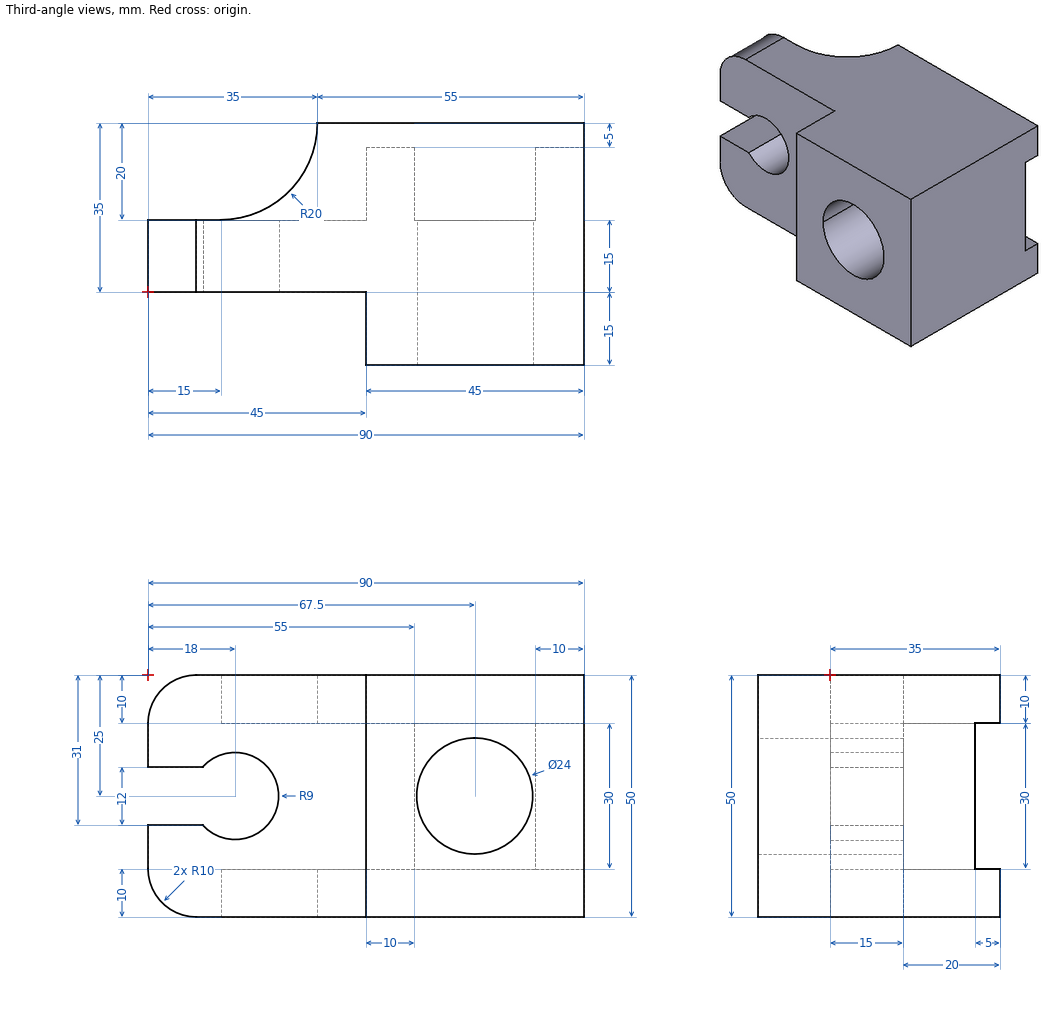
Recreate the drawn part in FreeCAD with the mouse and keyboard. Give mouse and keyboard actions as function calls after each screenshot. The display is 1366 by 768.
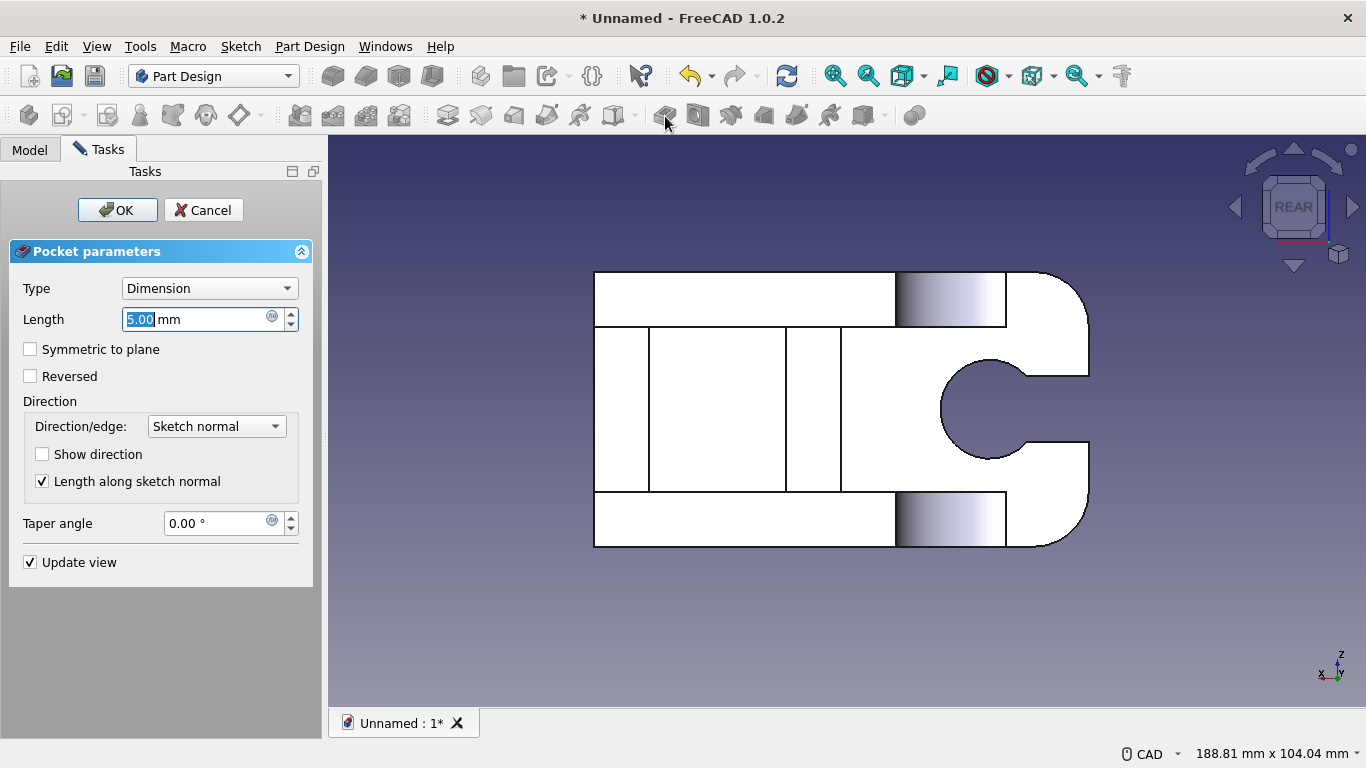
text(5)
key(Tab)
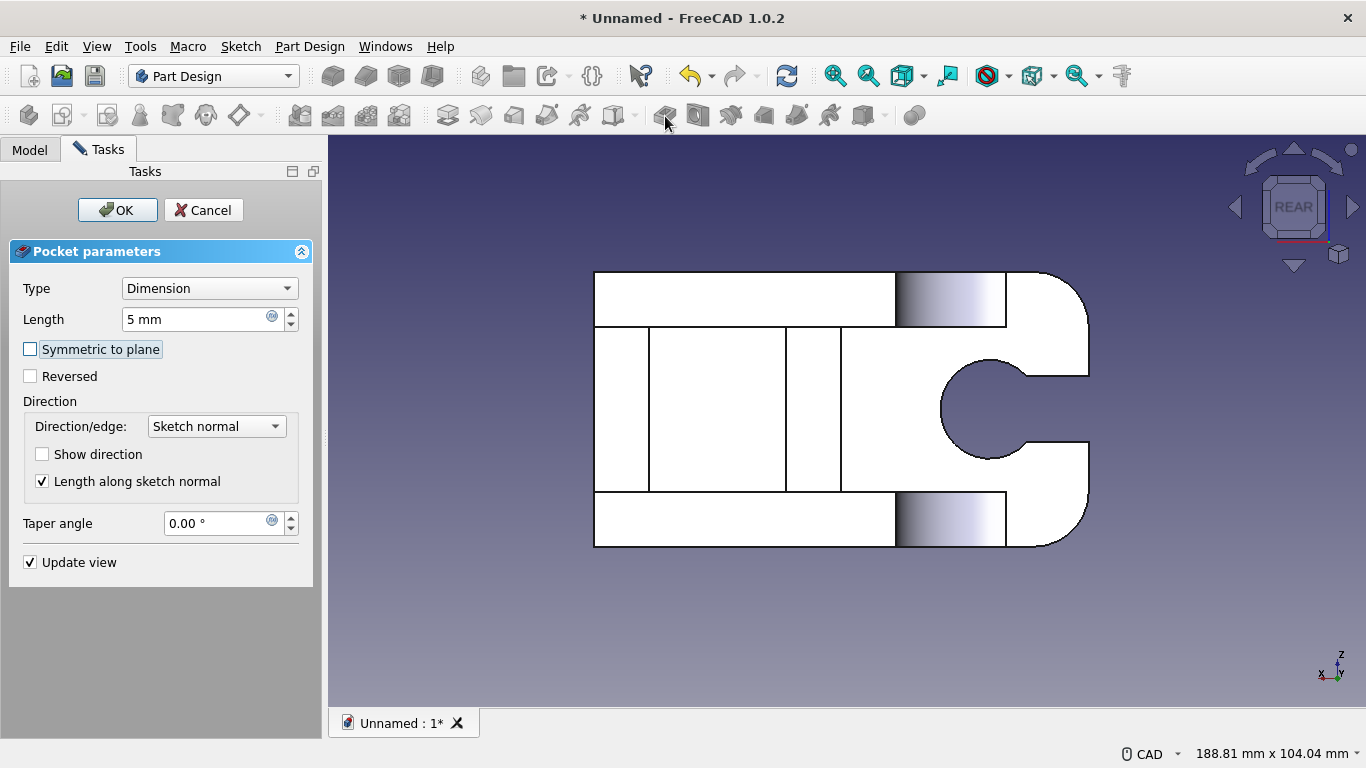
click(118, 210)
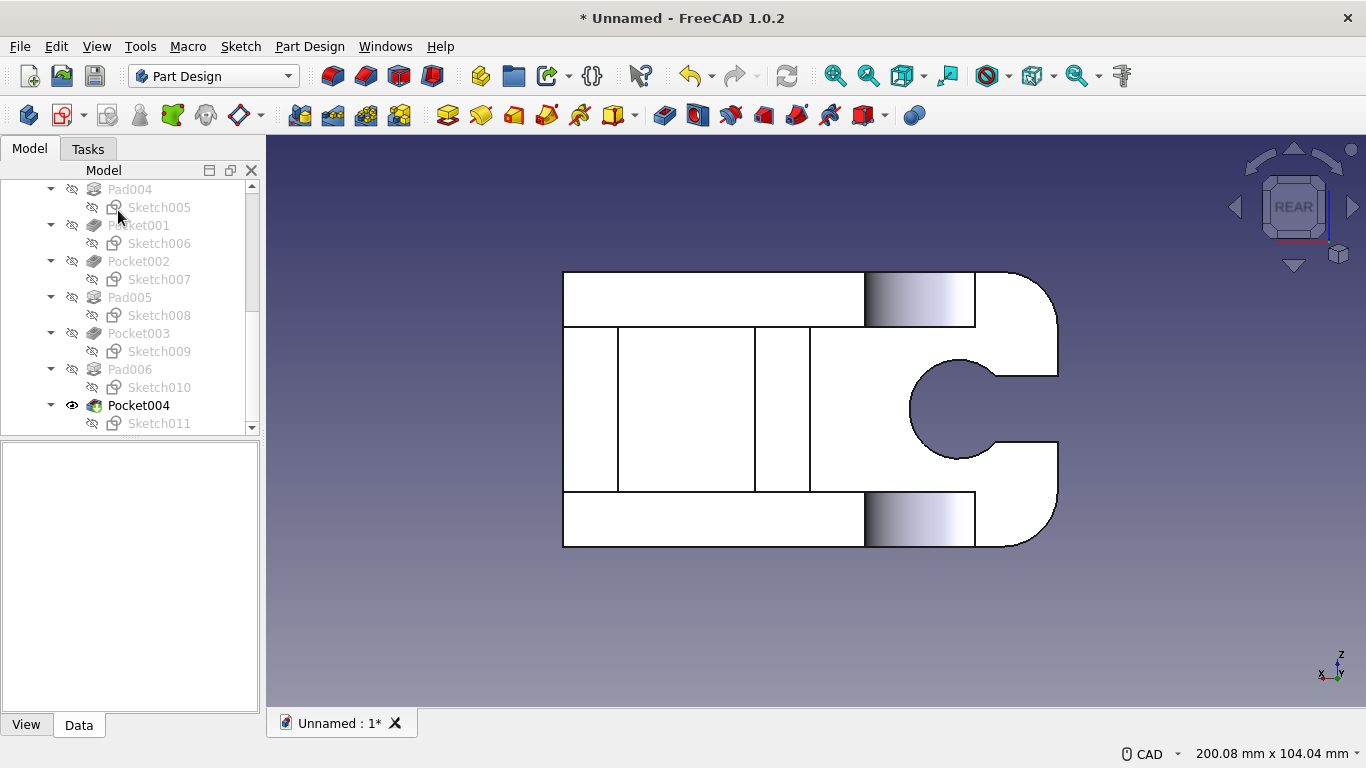
click(863, 408)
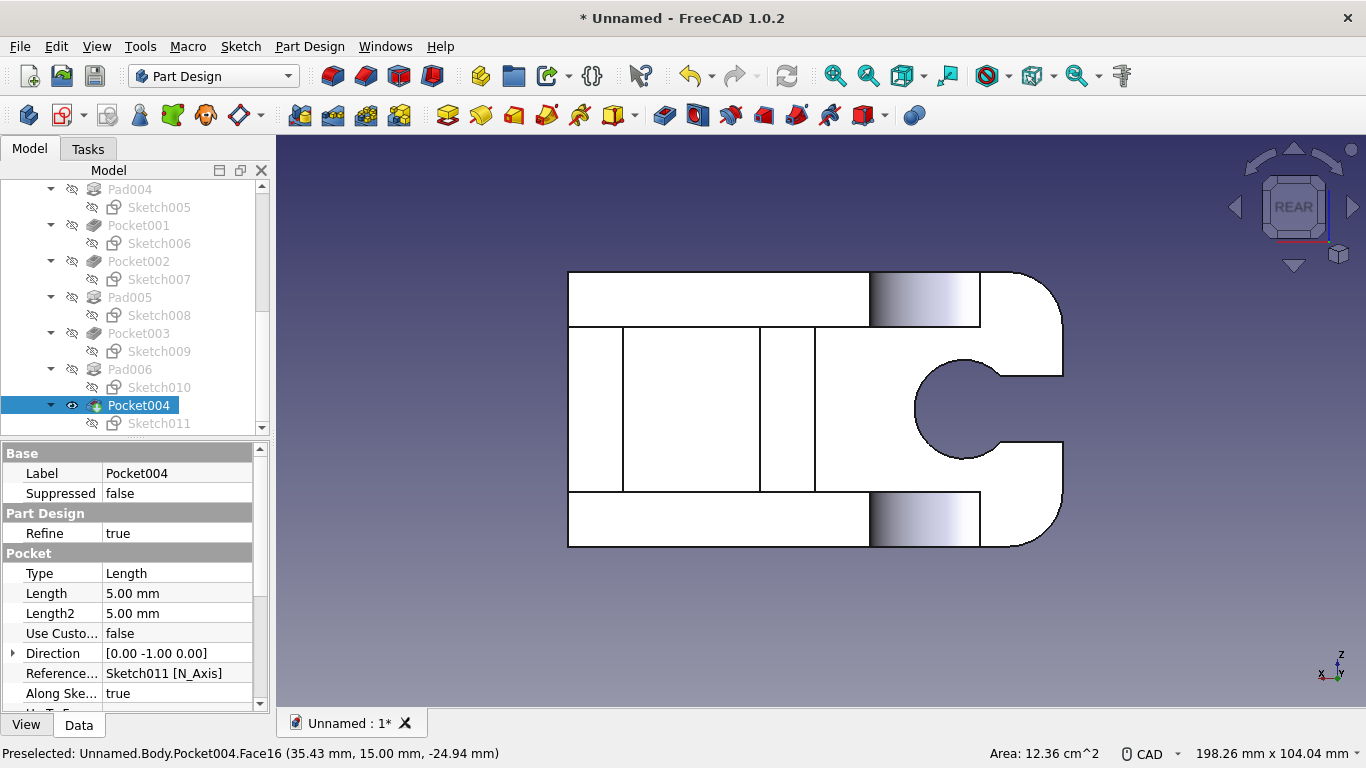
click(62, 116)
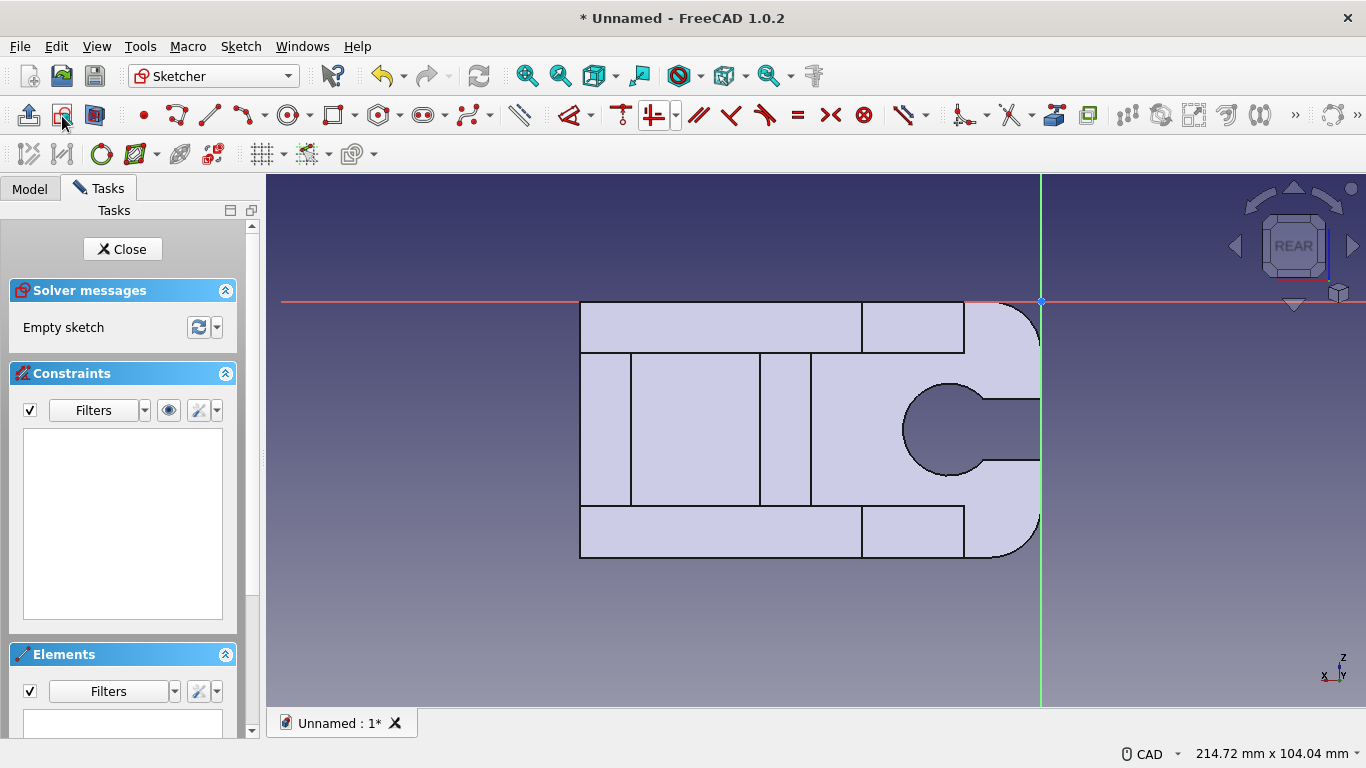
scroll(665, 423, up, 5)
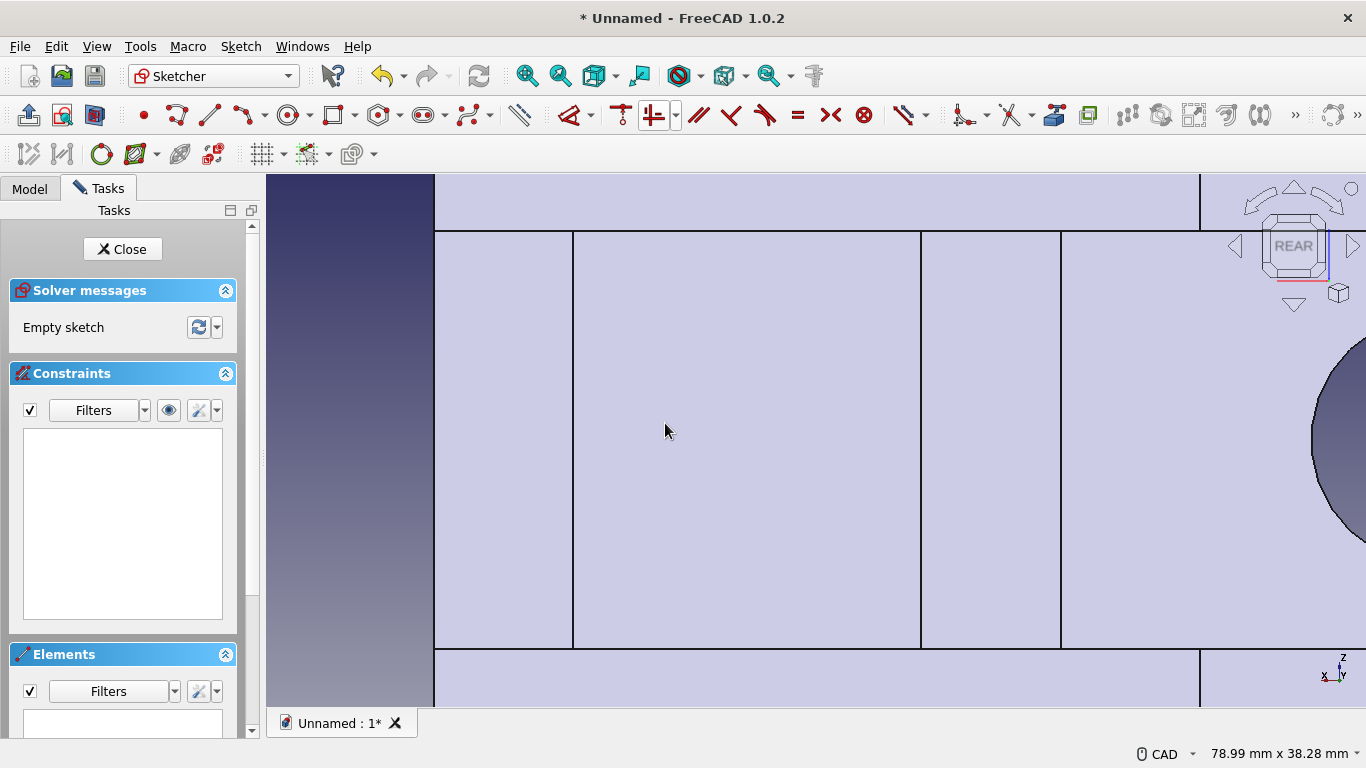
click(288, 116)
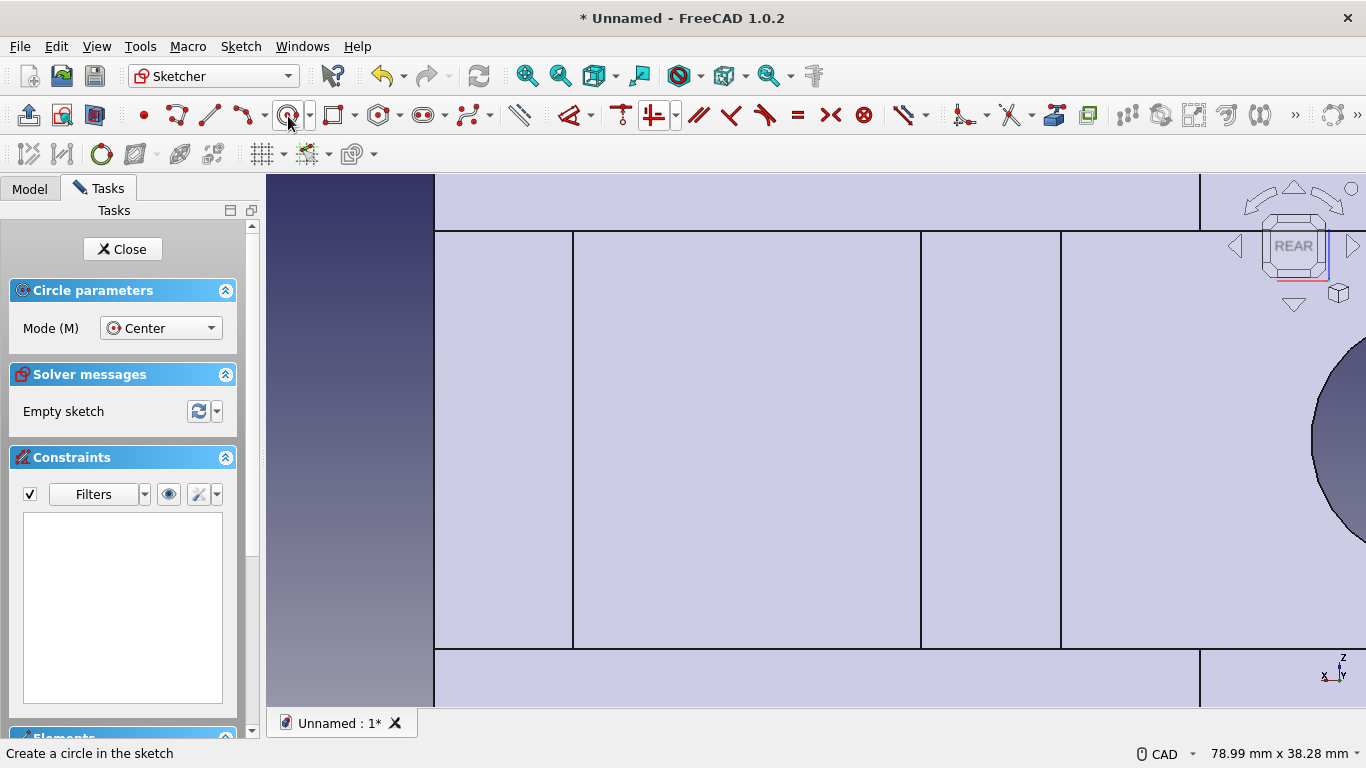
click(747, 440)
click(865, 322)
key(Escape)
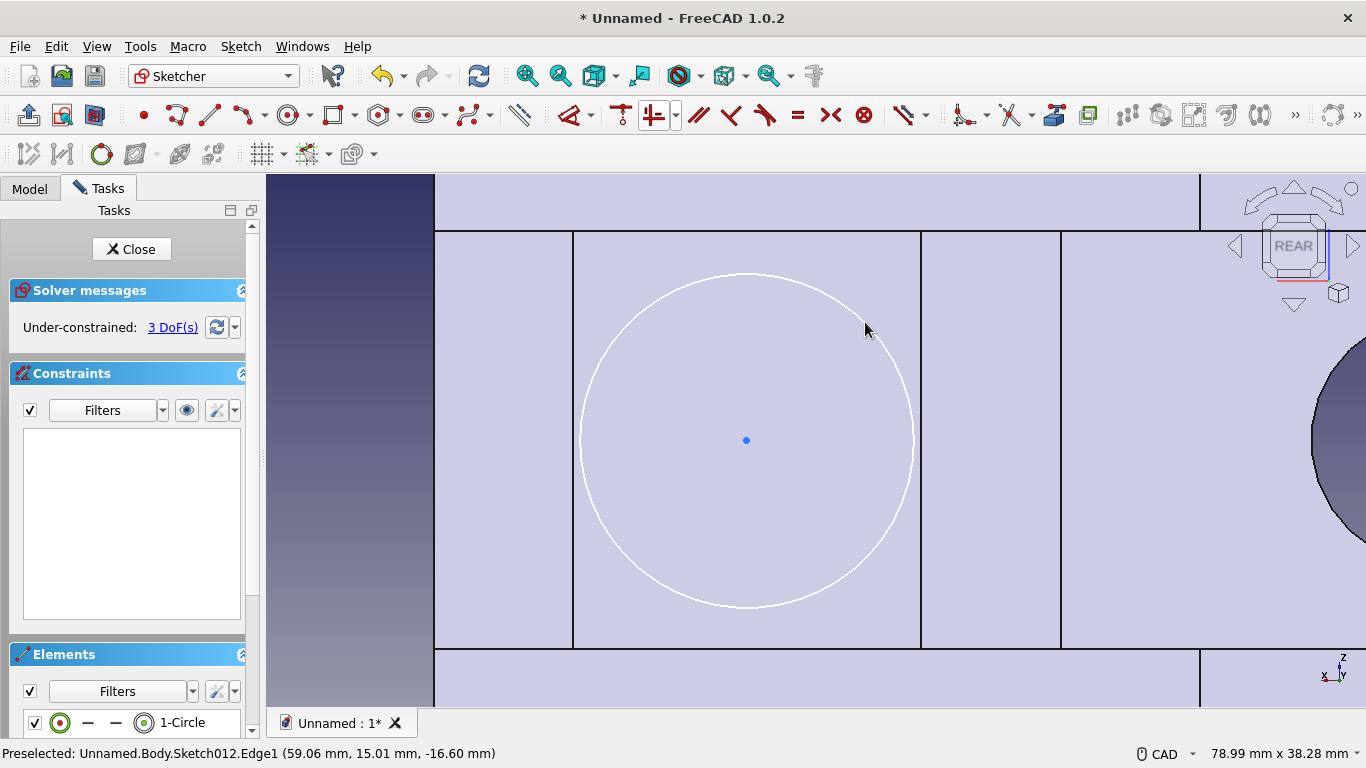
click(568, 116)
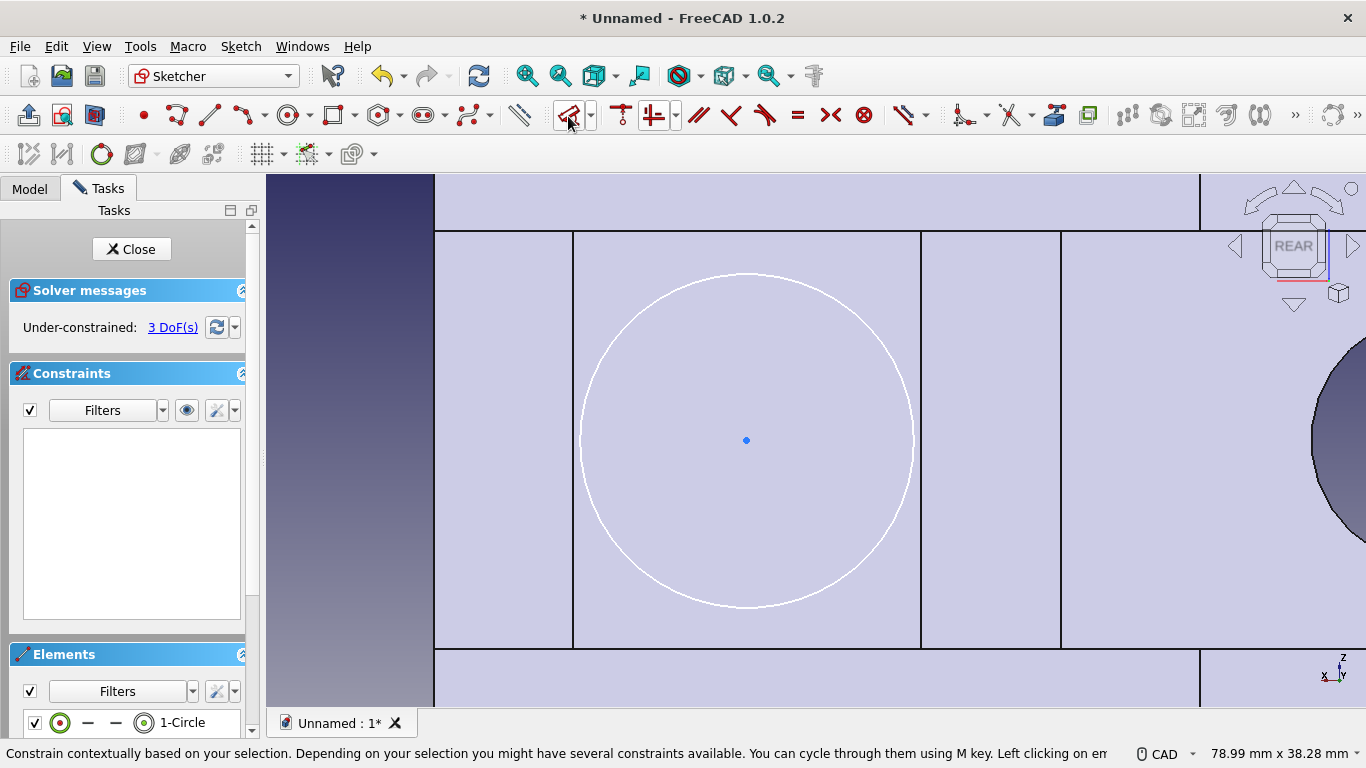
click(865, 323)
click(888, 300)